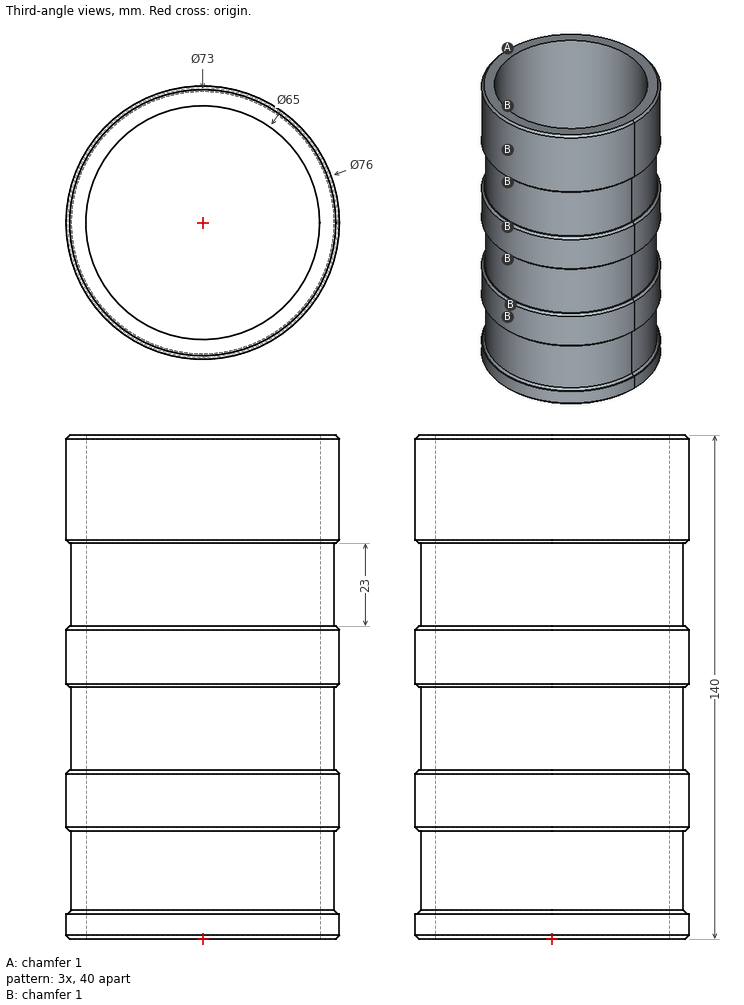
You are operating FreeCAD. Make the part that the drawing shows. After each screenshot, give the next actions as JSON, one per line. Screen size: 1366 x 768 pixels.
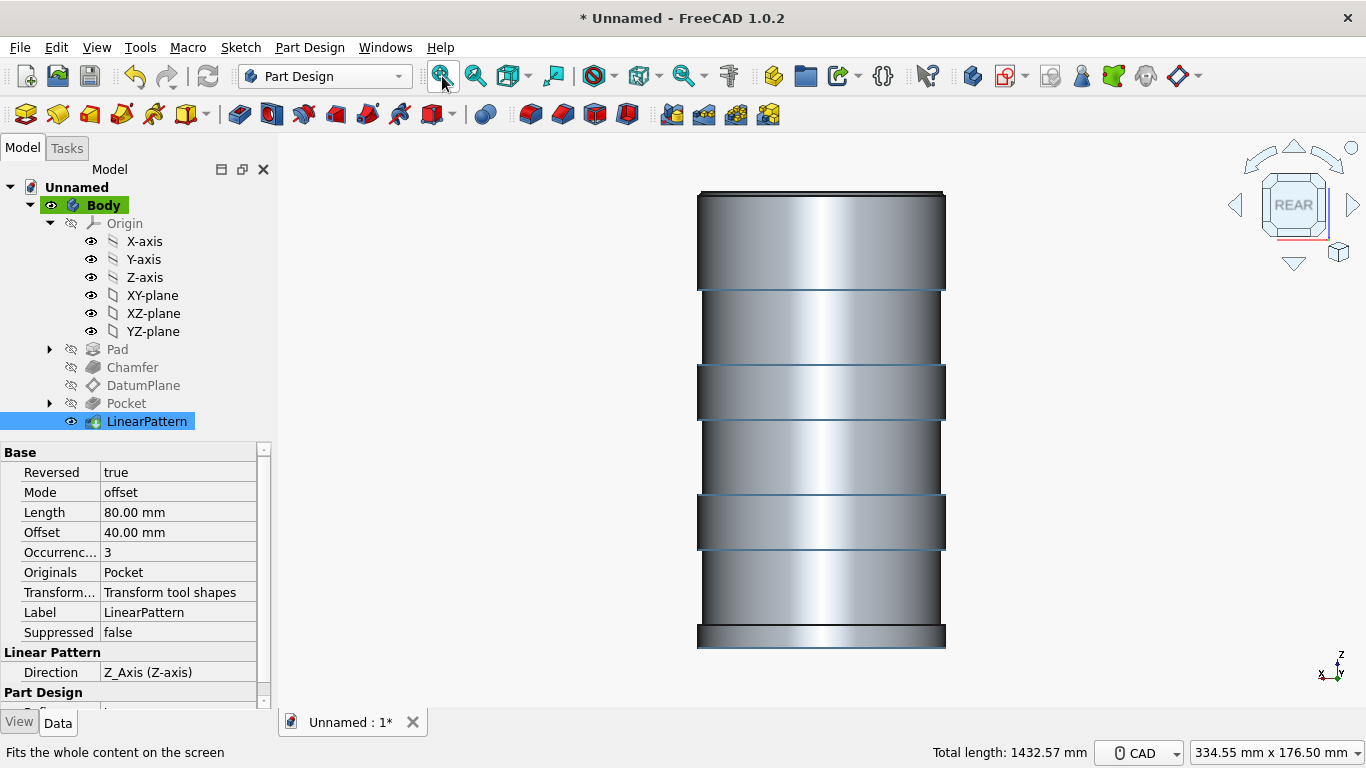
{"action": "key", "text": "6"}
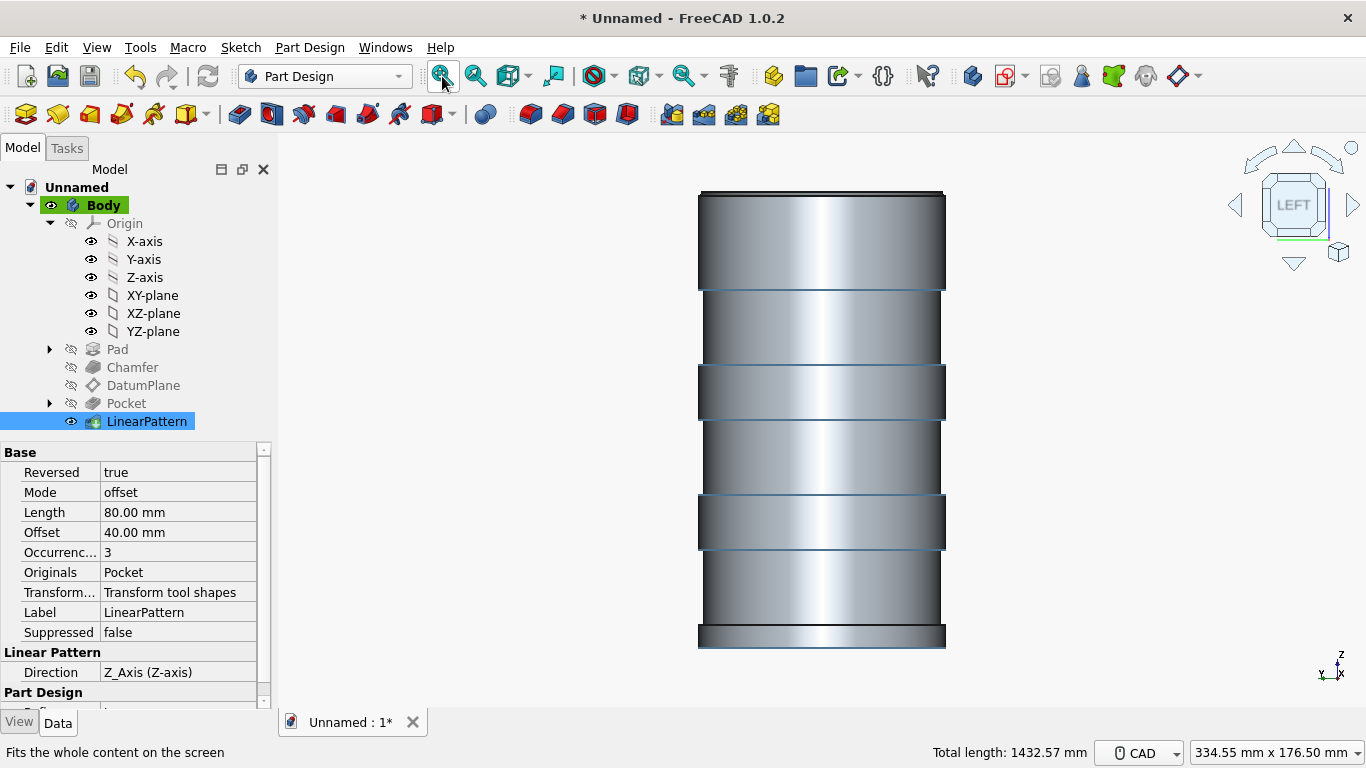
{"action": "key", "text": "v 3"}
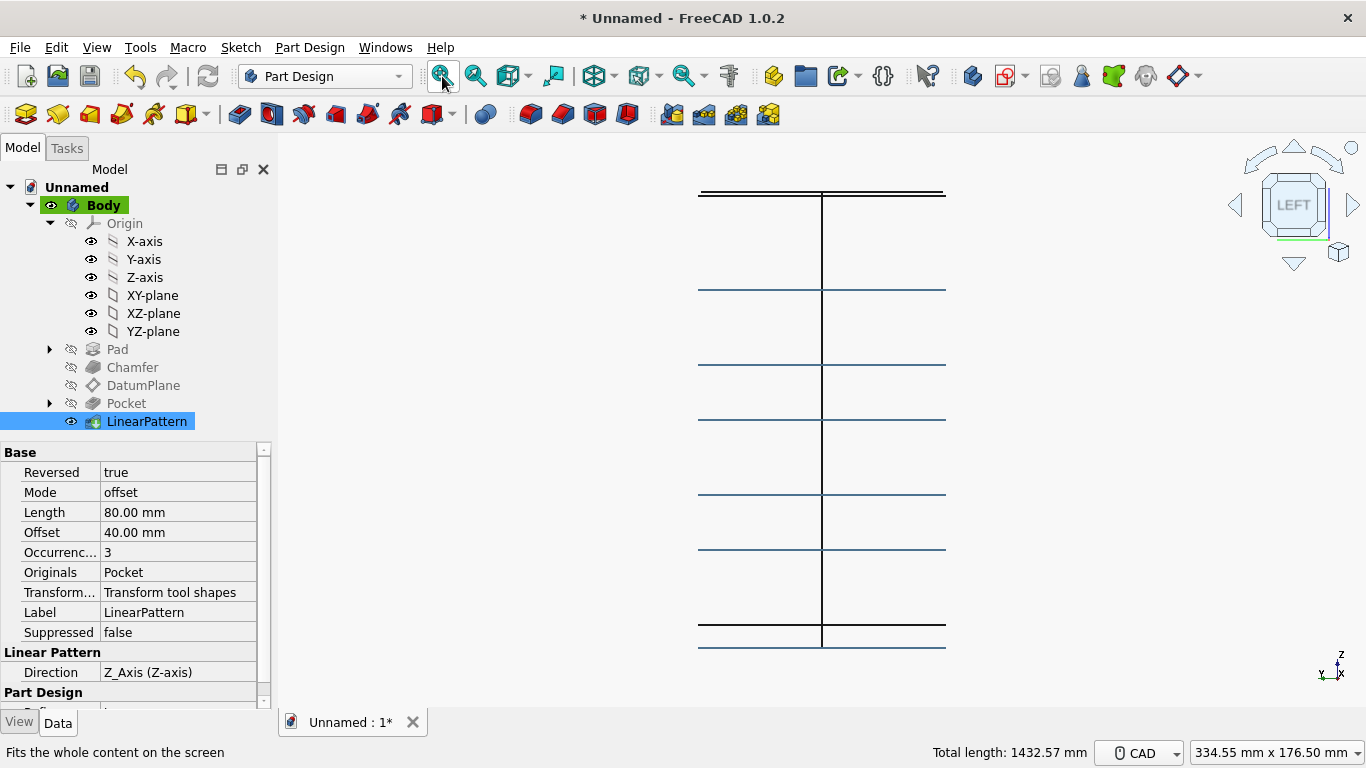
{"action": "key", "text": "0"}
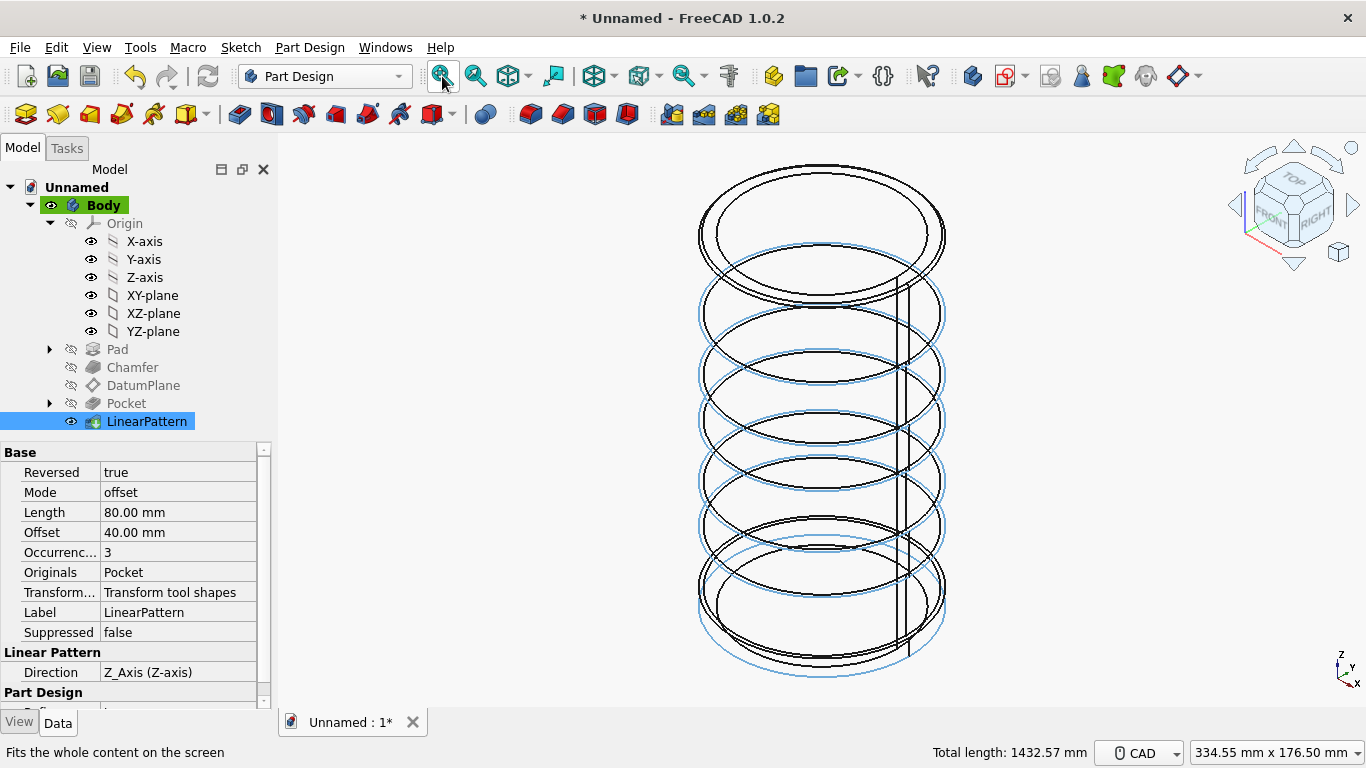
{"action": "key", "text": "v f"}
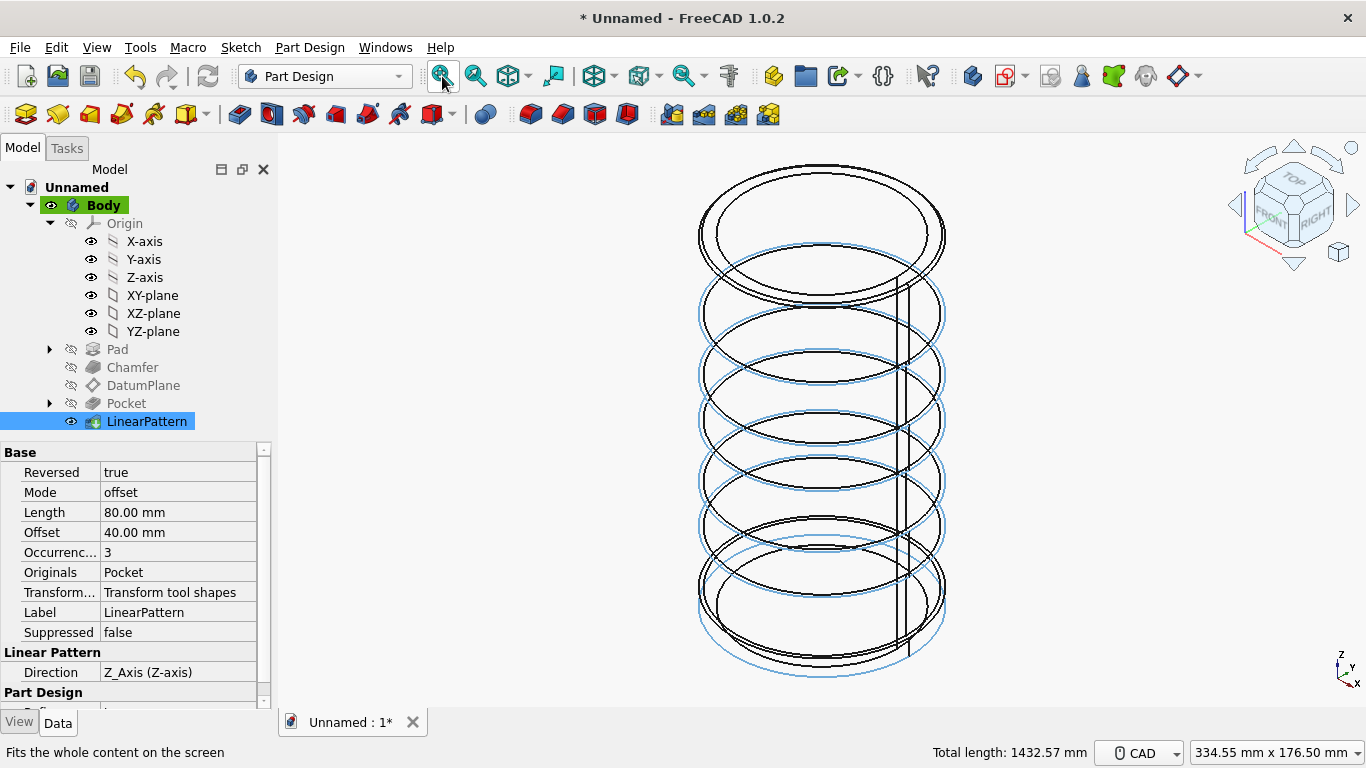
{"action": "left_click", "coordinate": [803, 519], "text": "ctrl"}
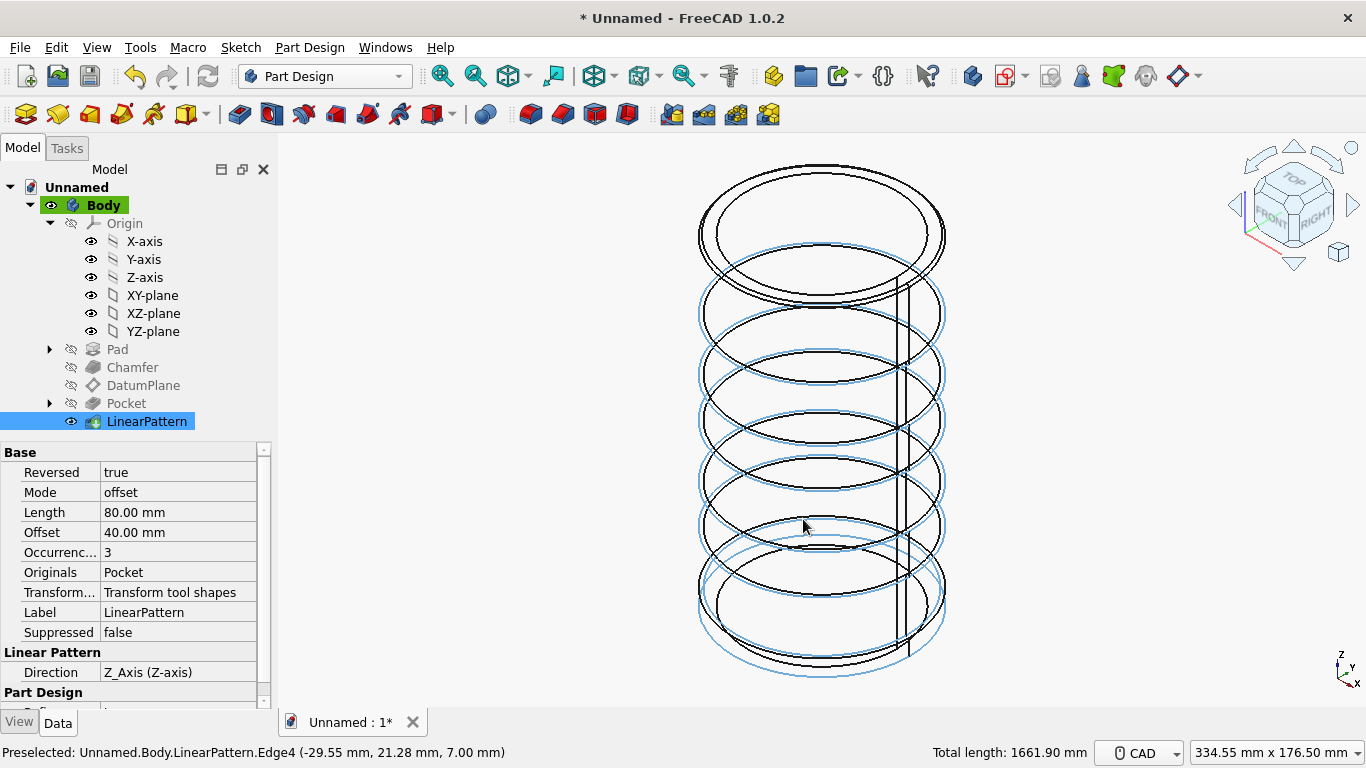
{"action": "key", "text": "v 1"}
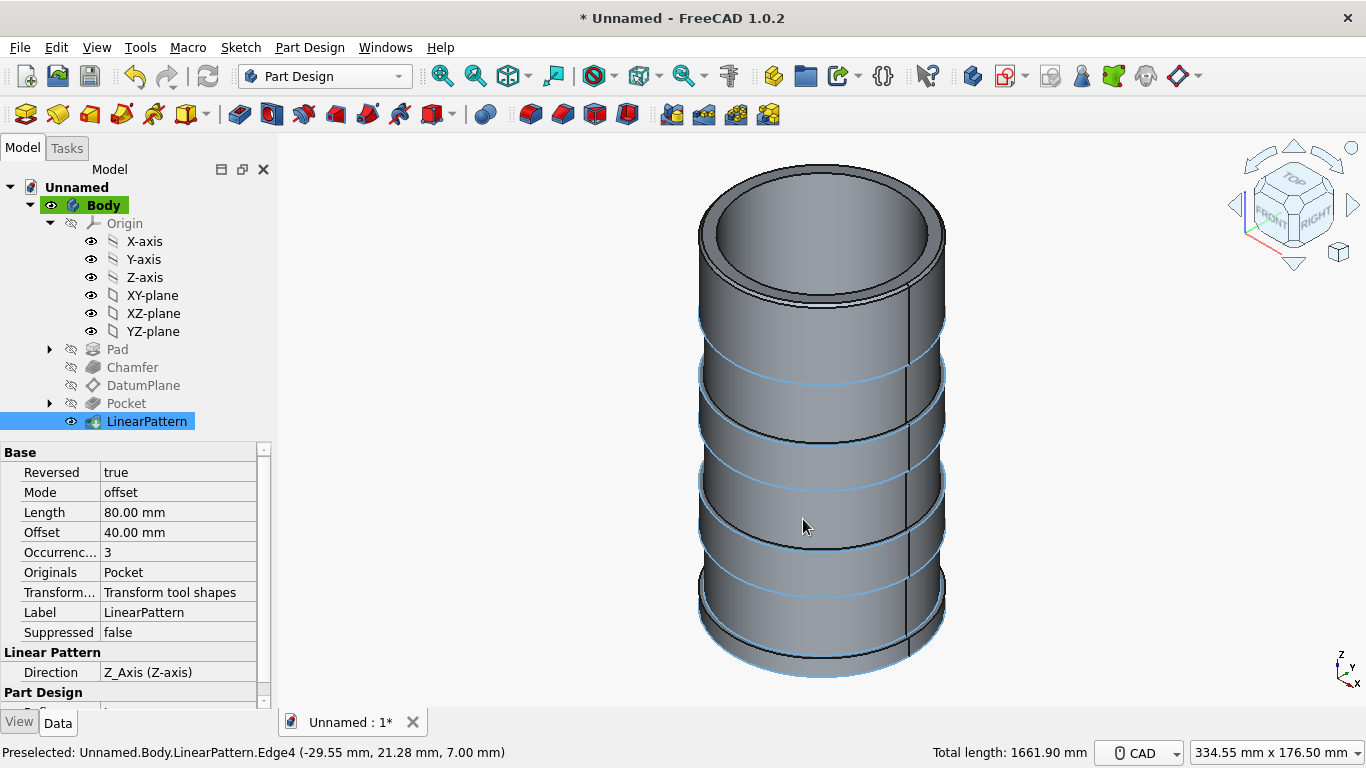
{"action": "left_click", "coordinate": [564, 114]}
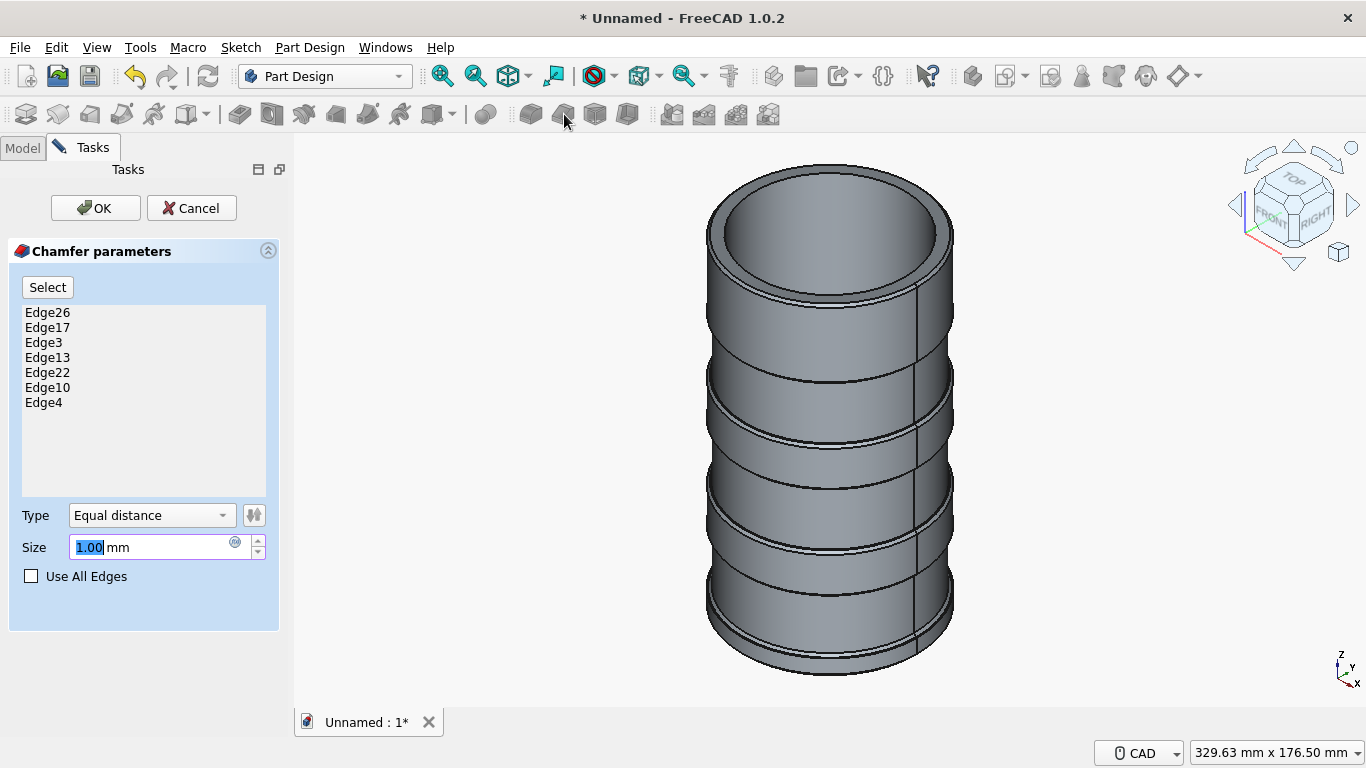
{"action": "type", "text": "1"}
{"action": "key", "text": "Tab"}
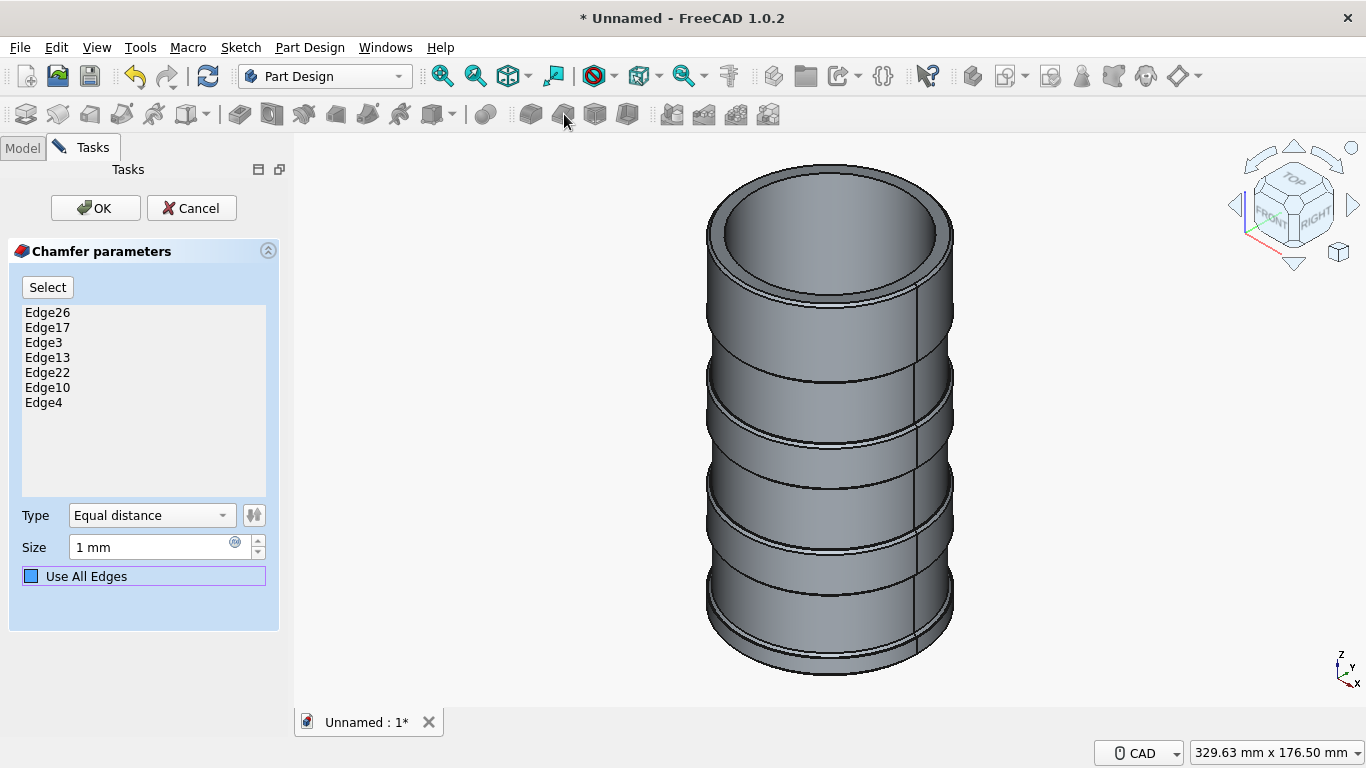
{"action": "left_click", "coordinate": [96, 208]}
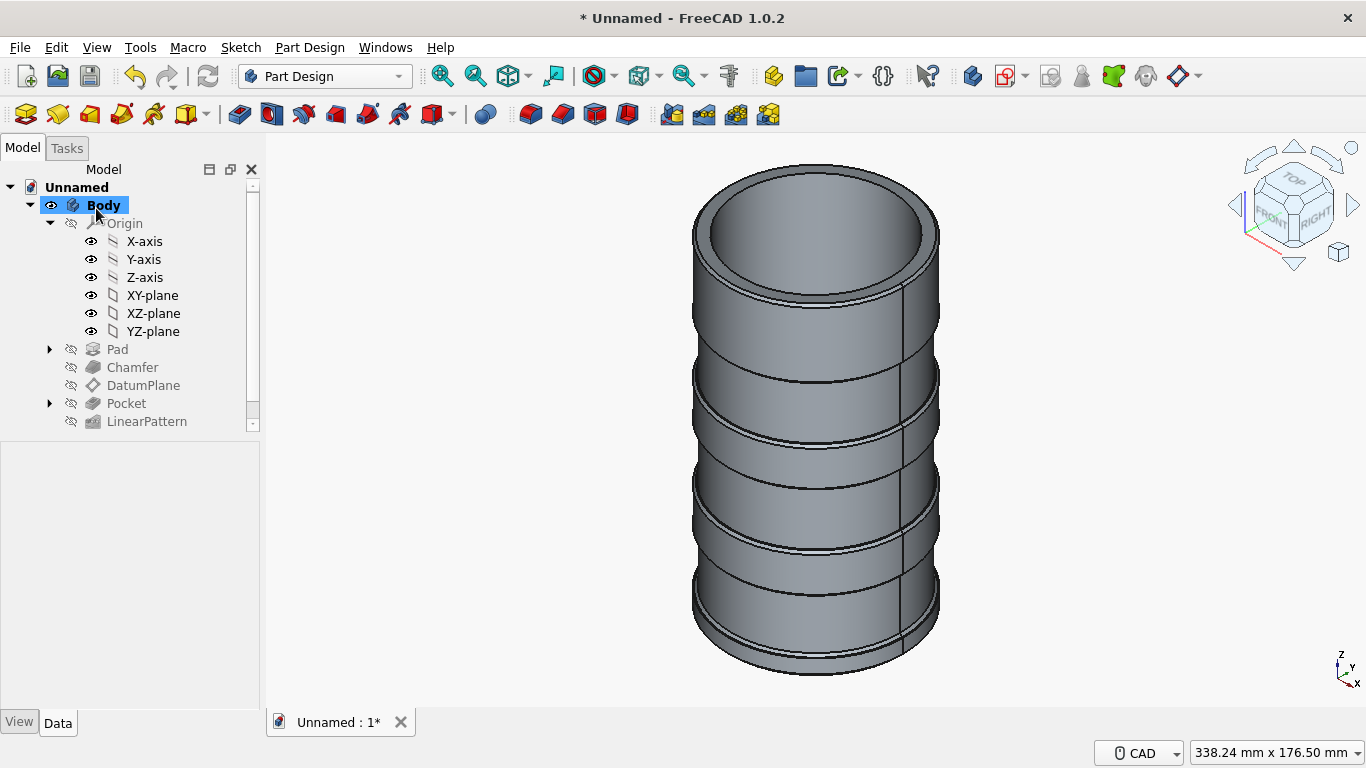
{"action": "key", "text": "v f"}